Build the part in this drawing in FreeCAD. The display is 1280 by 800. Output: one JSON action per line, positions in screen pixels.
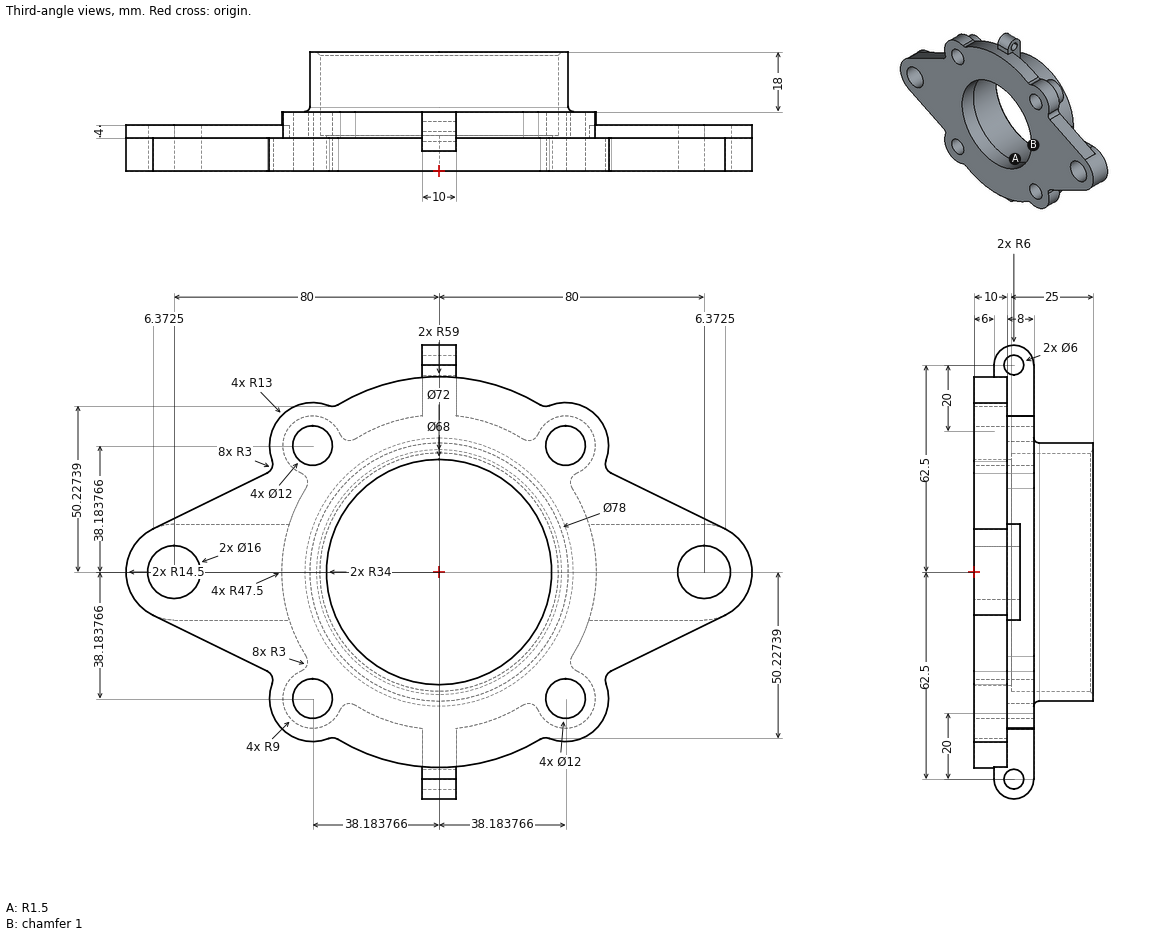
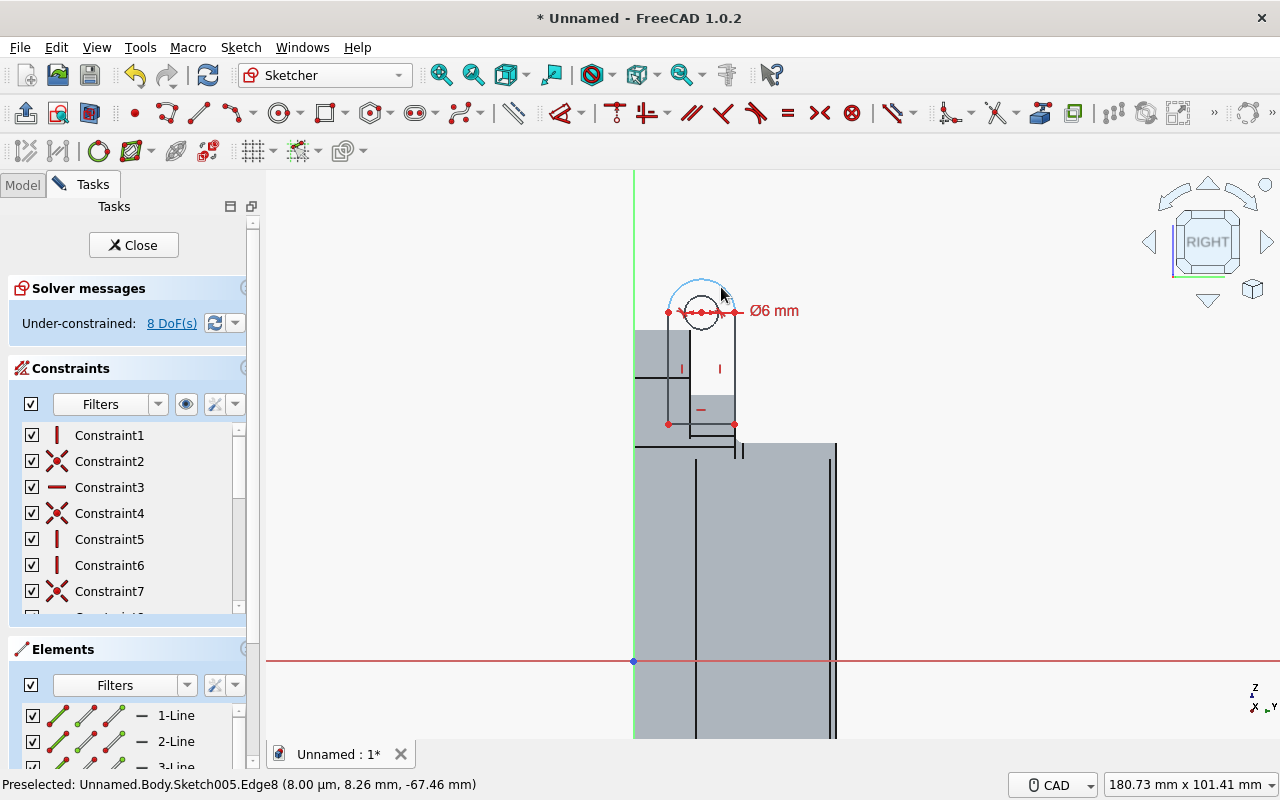
{"action": "left_click", "coordinate": [721, 286]}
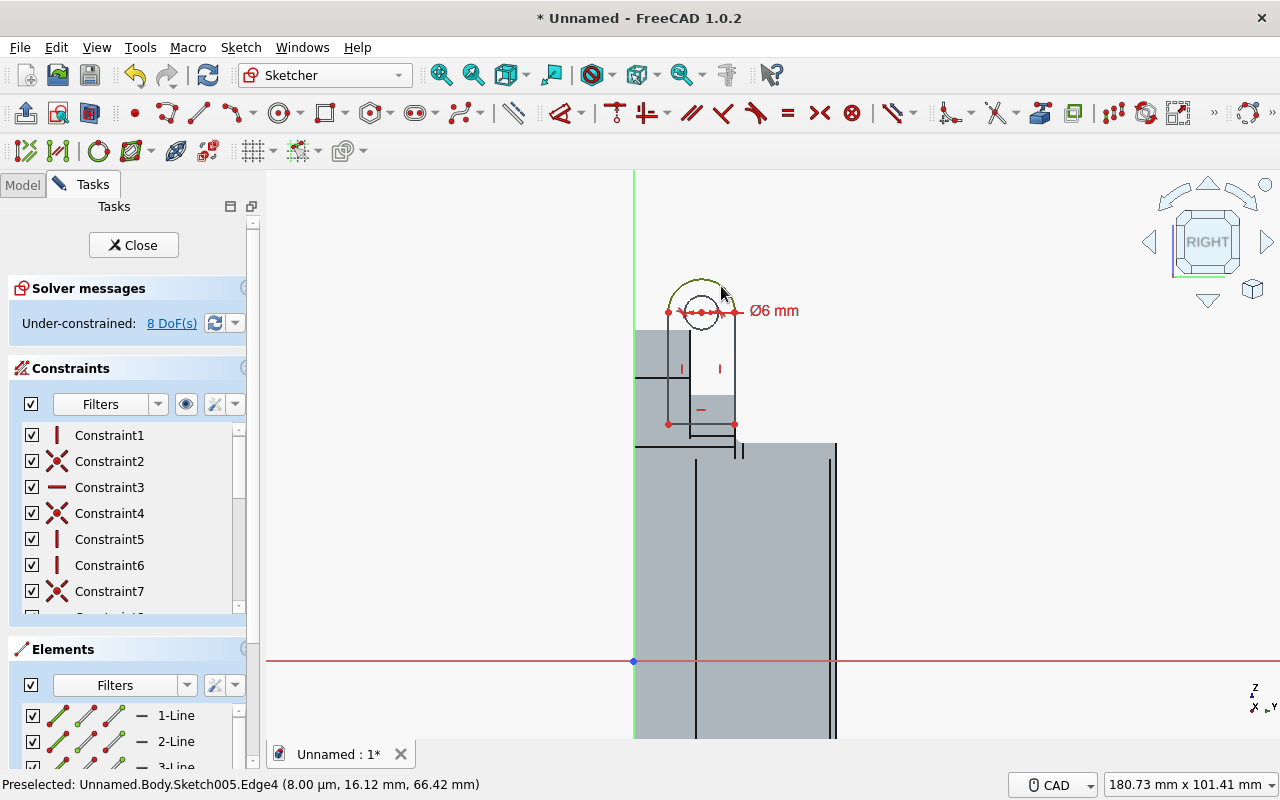
{"action": "scroll", "coordinate": [721, 286], "scroll_direction": "down", "scroll_amount": 4}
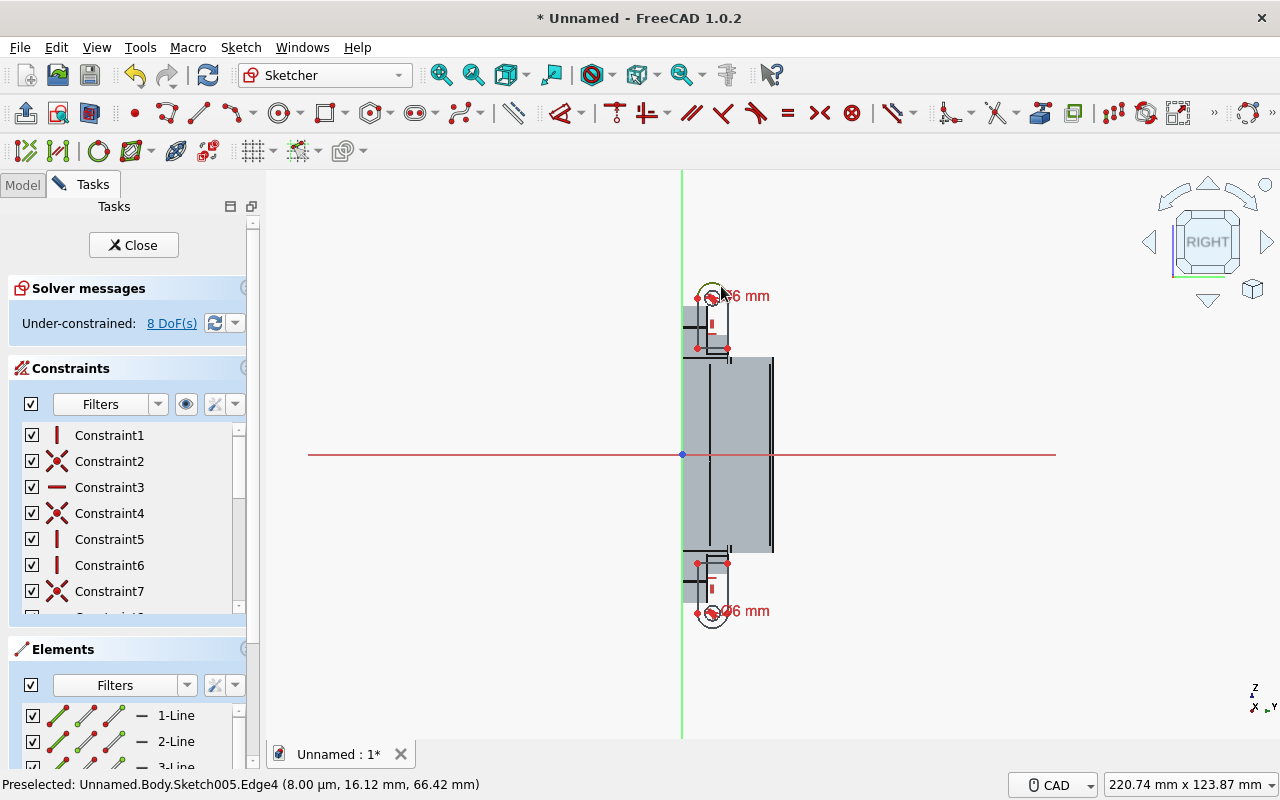
{"action": "scroll", "coordinate": [704, 625], "scroll_direction": "up", "scroll_amount": 4}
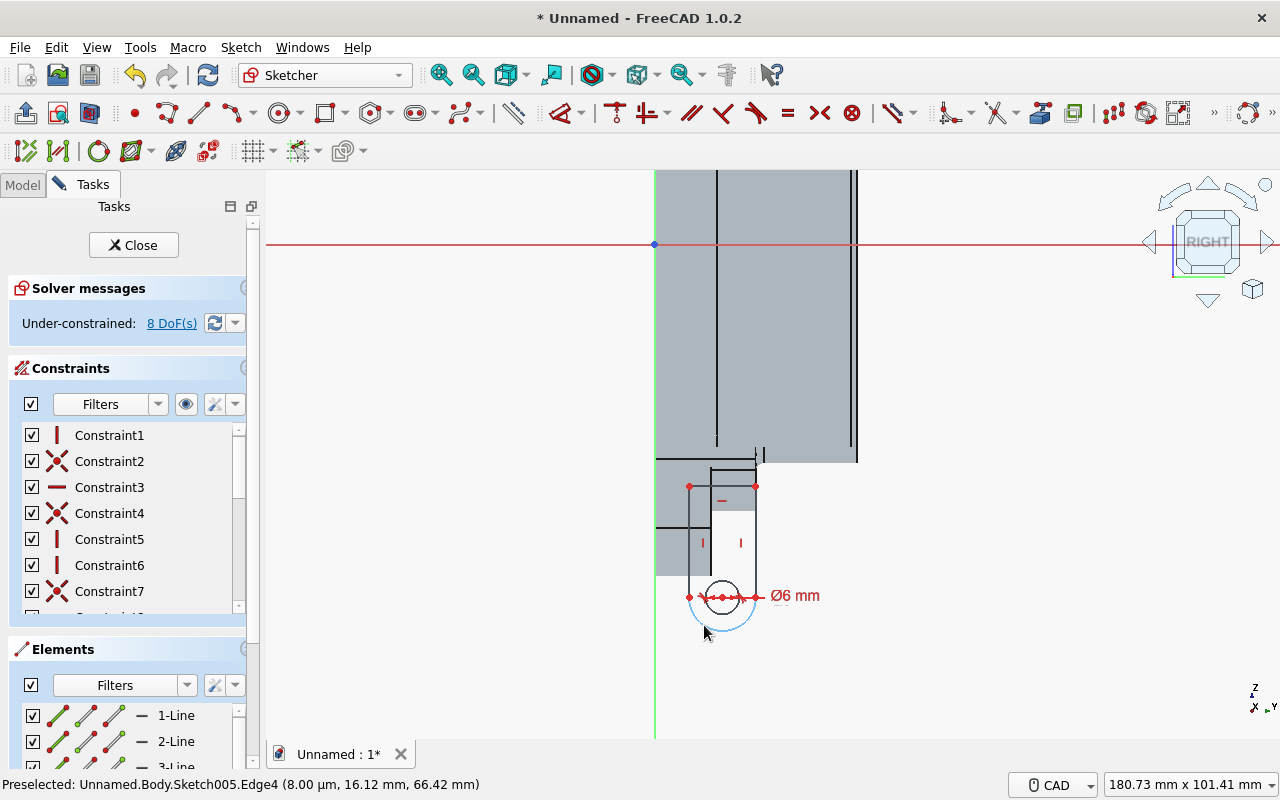
{"action": "left_click", "coordinate": [703, 625]}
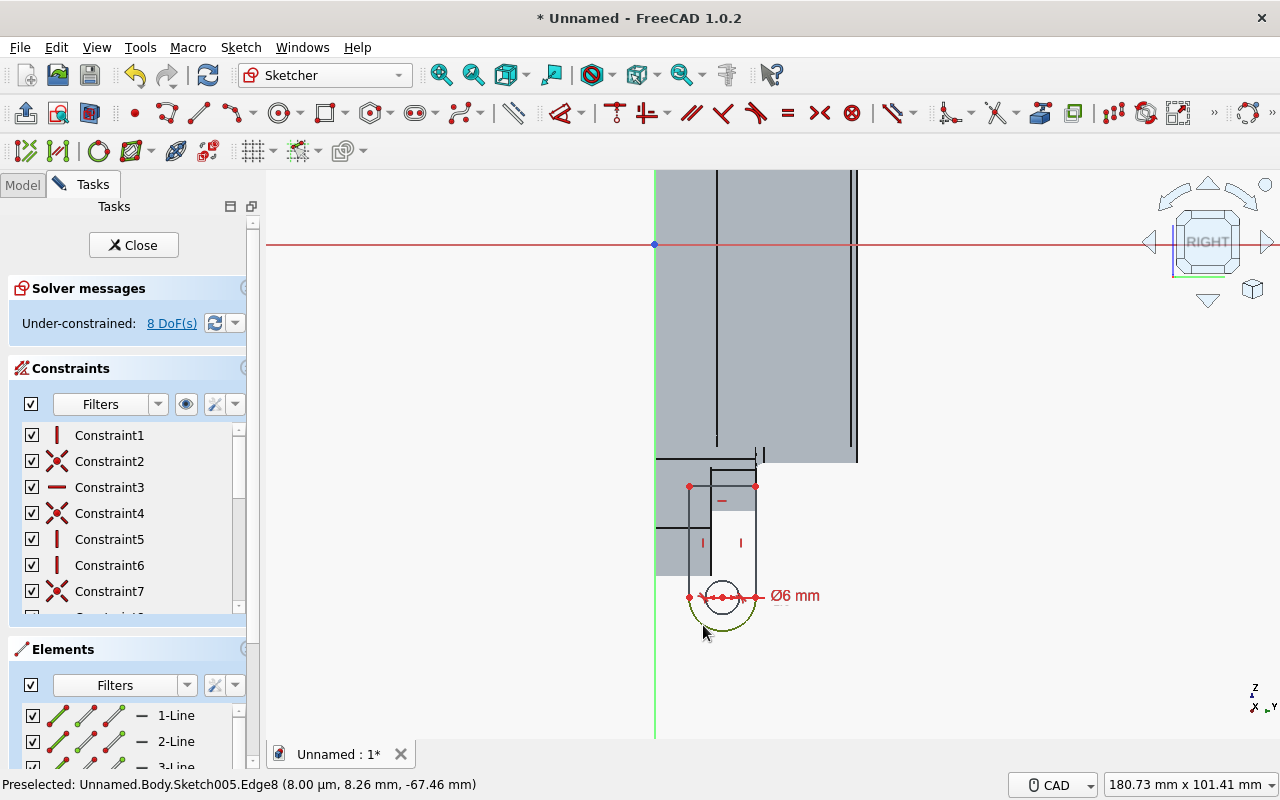
{"action": "left_click", "coordinate": [788, 114]}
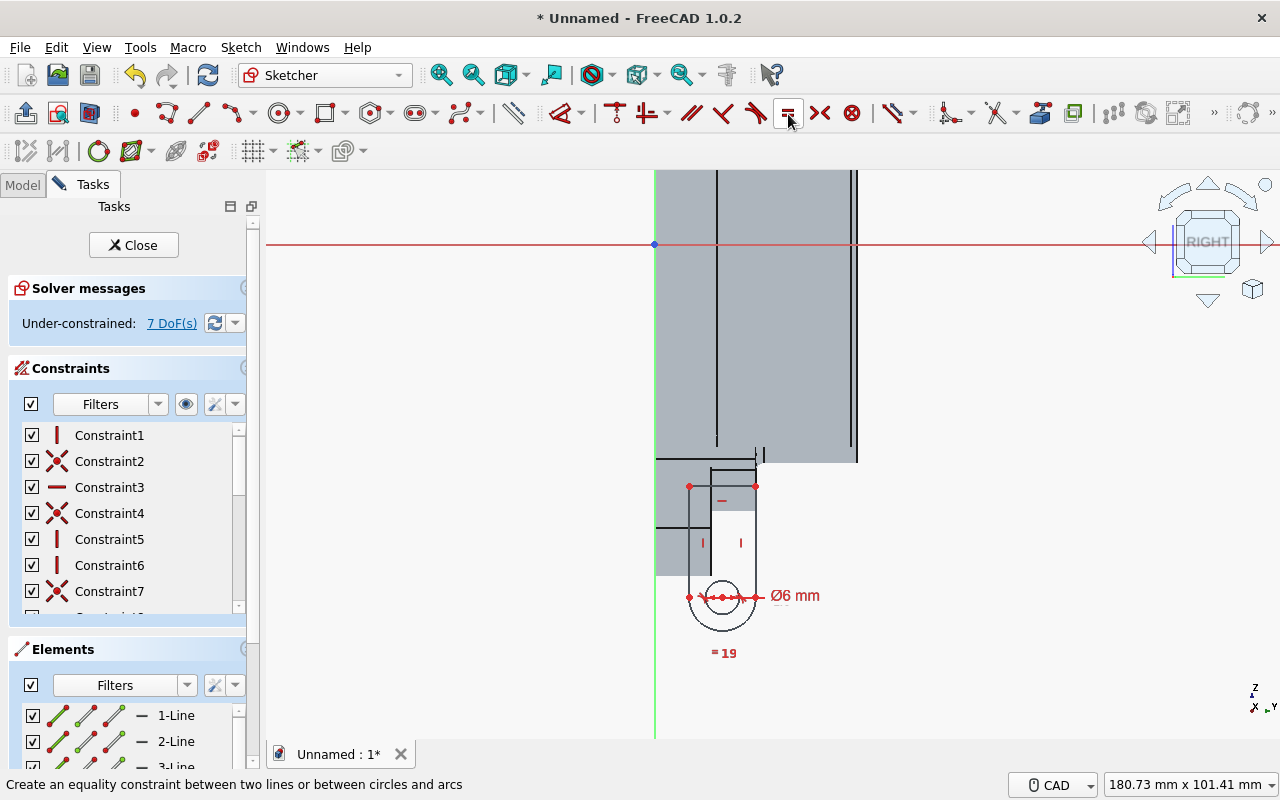
{"action": "left_click", "coordinate": [560, 114]}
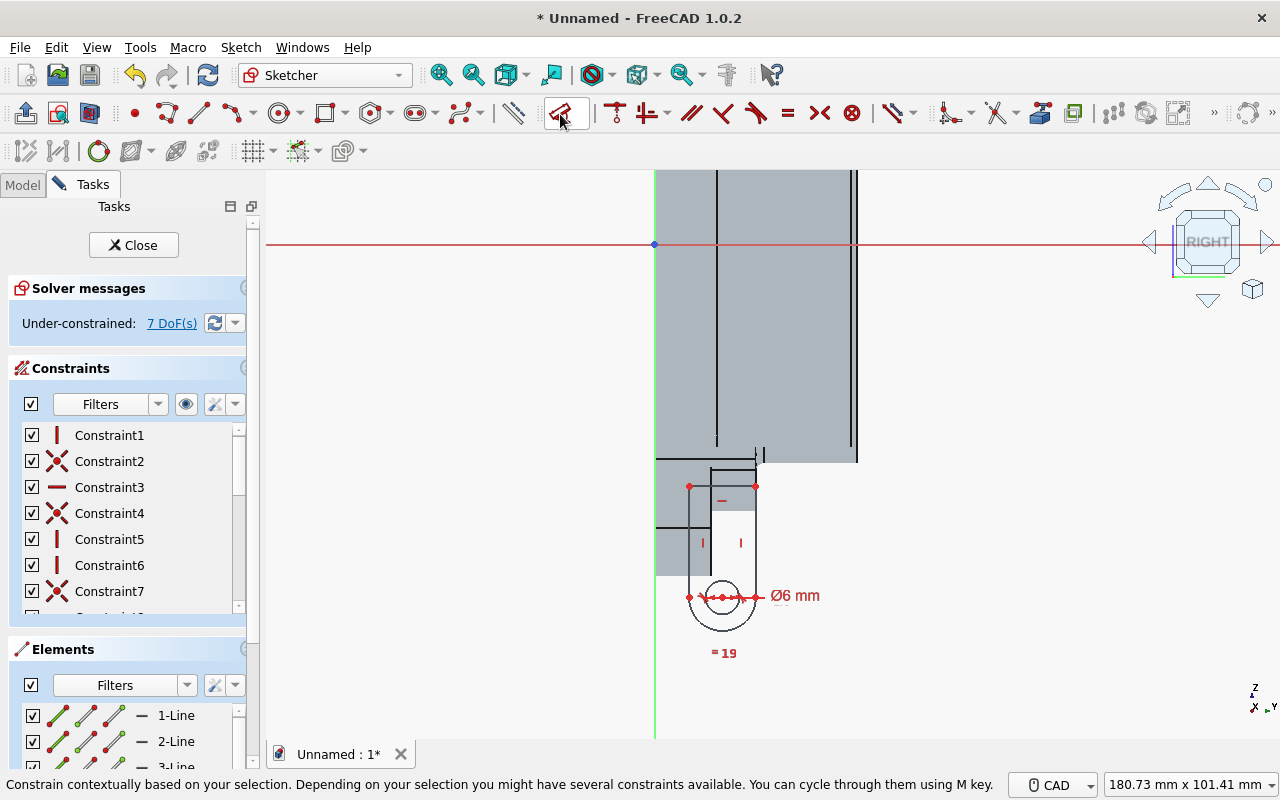
{"action": "scroll", "coordinate": [704, 626], "scroll_direction": "down", "scroll_amount": 4}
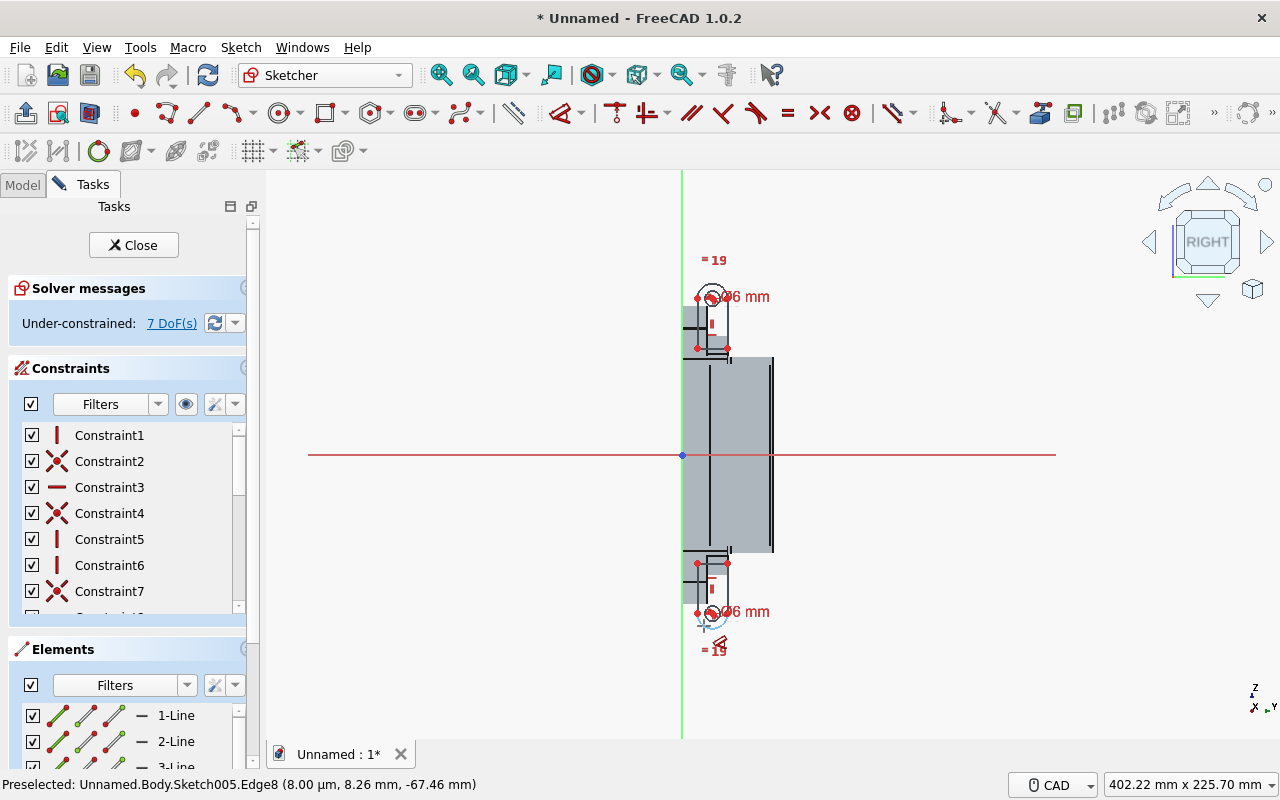
{"action": "scroll", "coordinate": [721, 287], "scroll_direction": "up", "scroll_amount": 5}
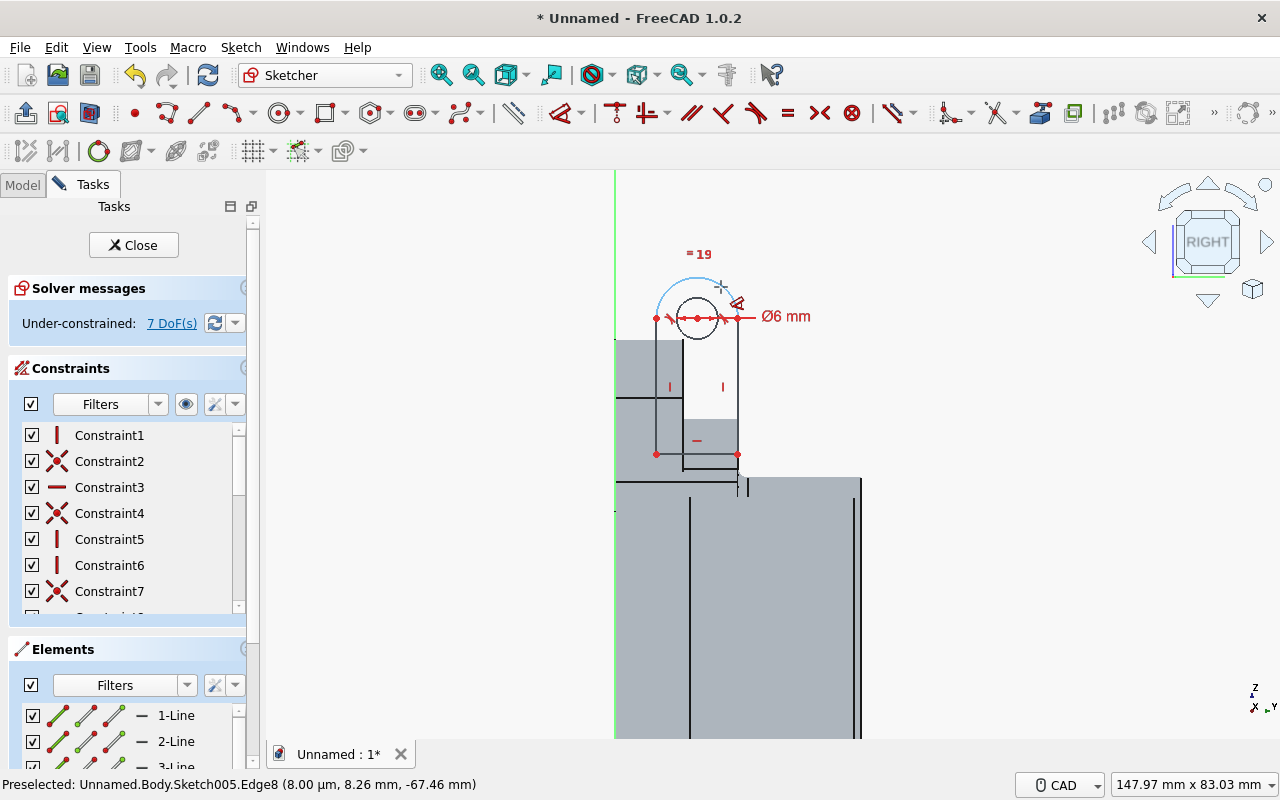
{"action": "left_click", "coordinate": [721, 285]}
{"action": "left_click", "coordinate": [740, 259]}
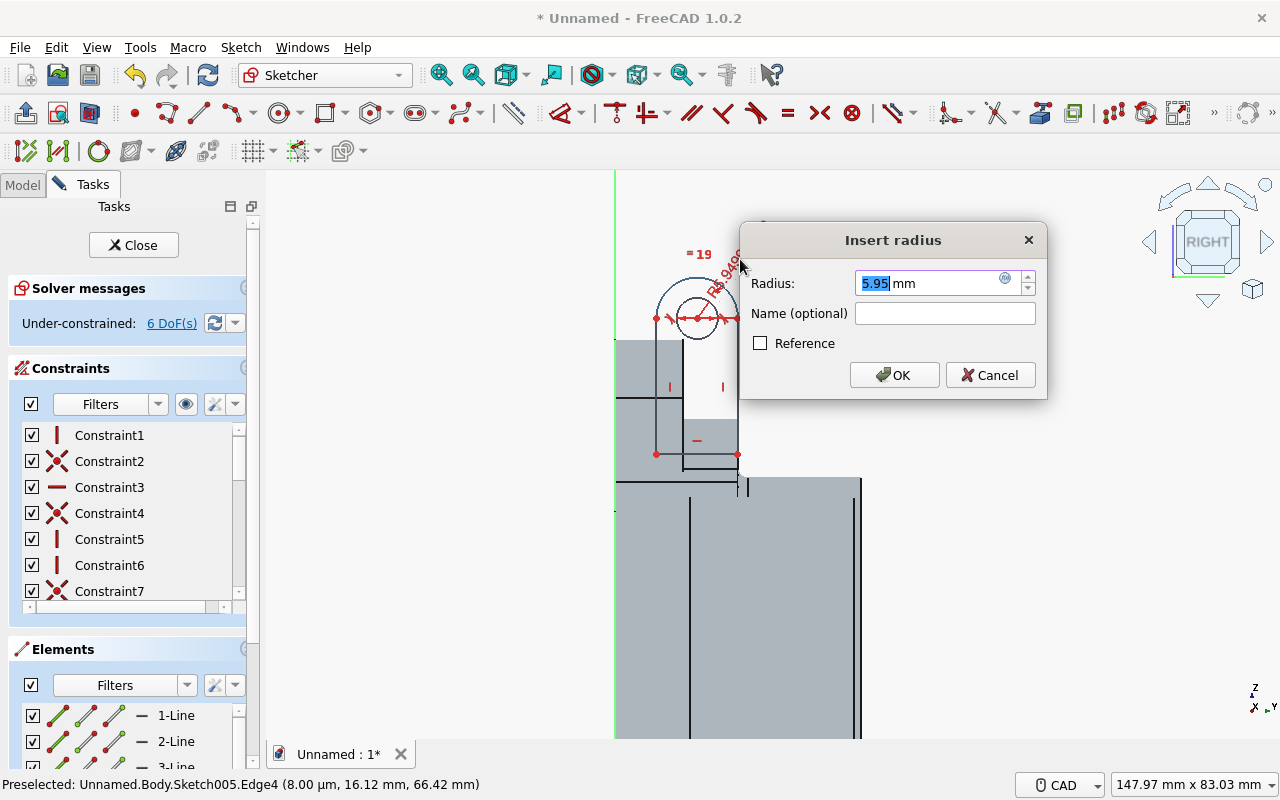
{"action": "type", "text": "6"}
{"action": "key", "text": "Return"}